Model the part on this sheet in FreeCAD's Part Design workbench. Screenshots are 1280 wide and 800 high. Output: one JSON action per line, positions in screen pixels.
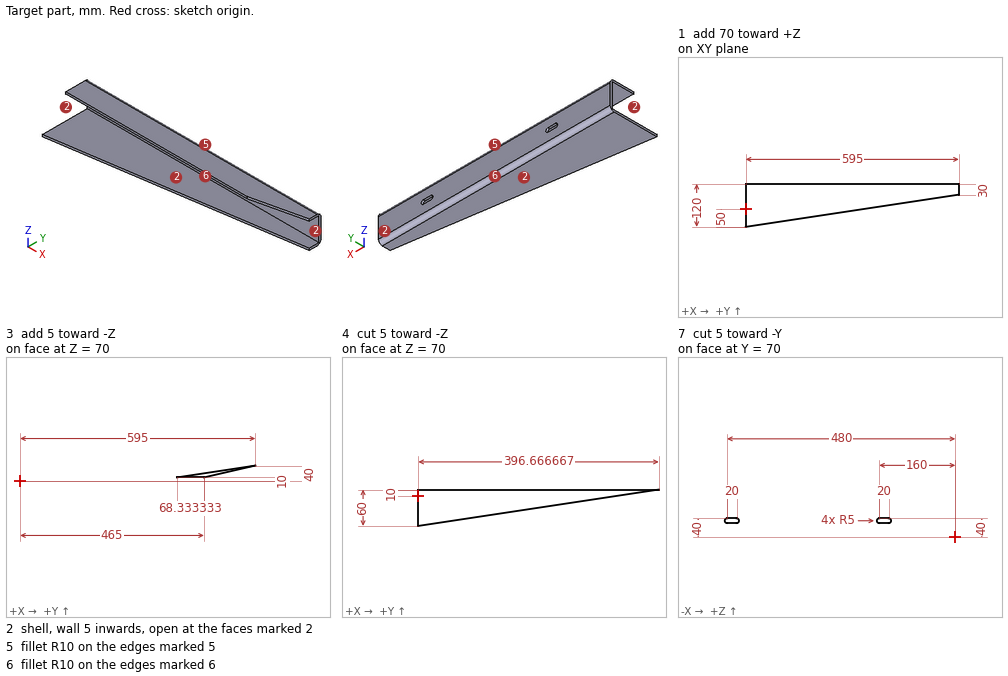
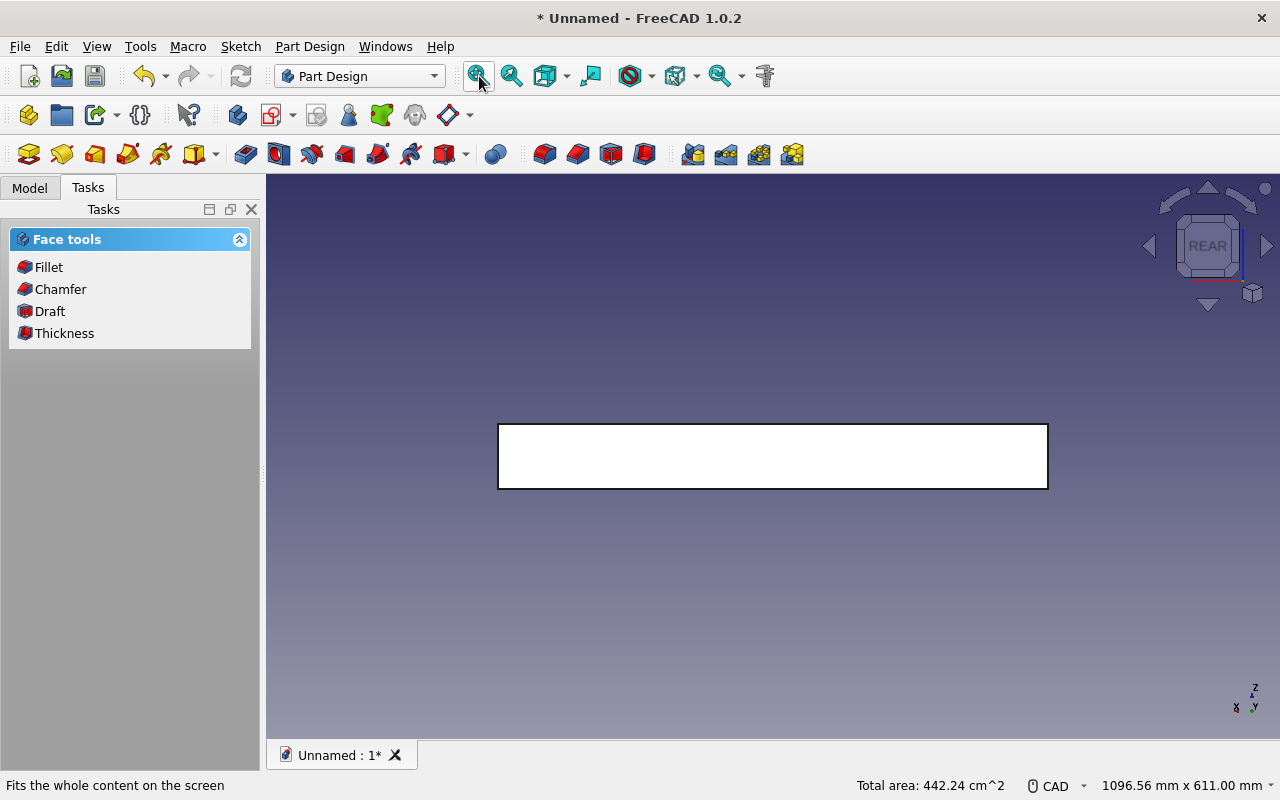
{"action": "key", "text": "6"}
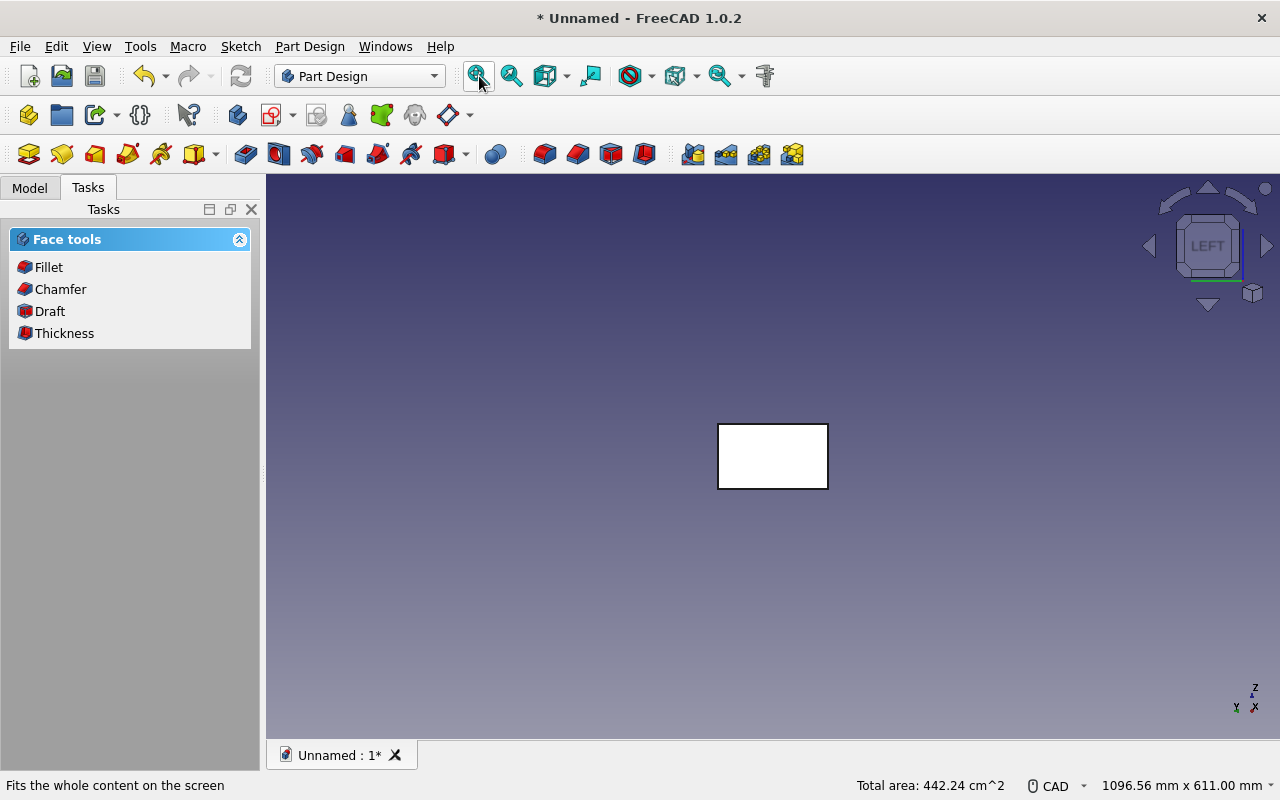
{"action": "key", "text": "v f"}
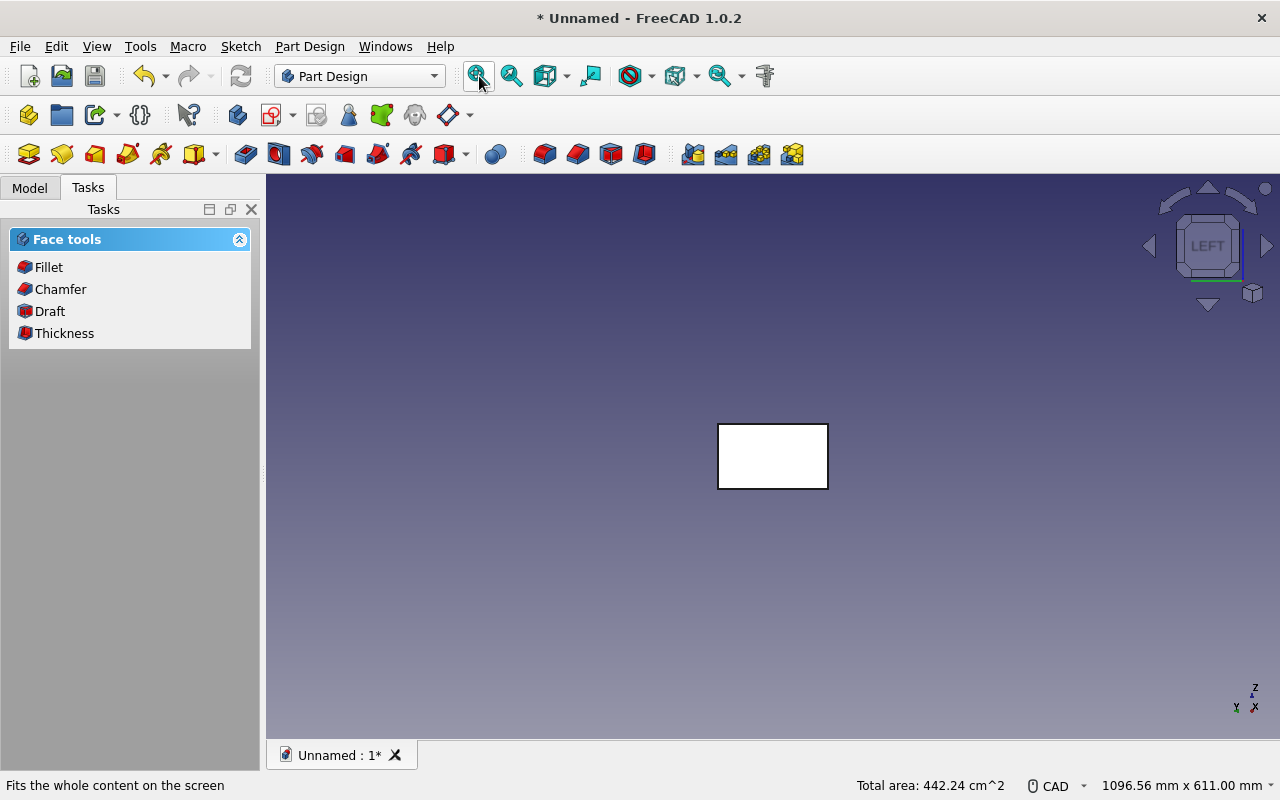
{"action": "left_click", "coordinate": [757, 455], "text": "ctrl"}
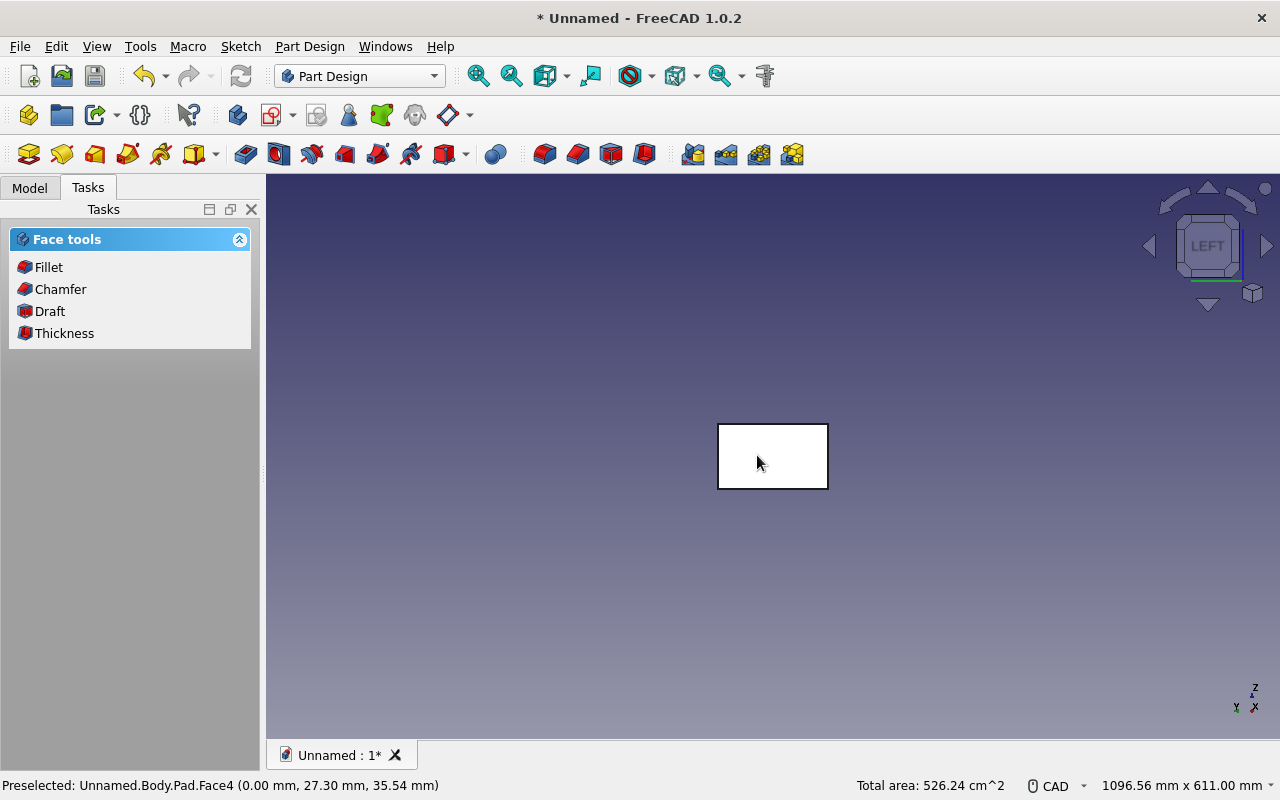
{"action": "left_click", "coordinate": [644, 154]}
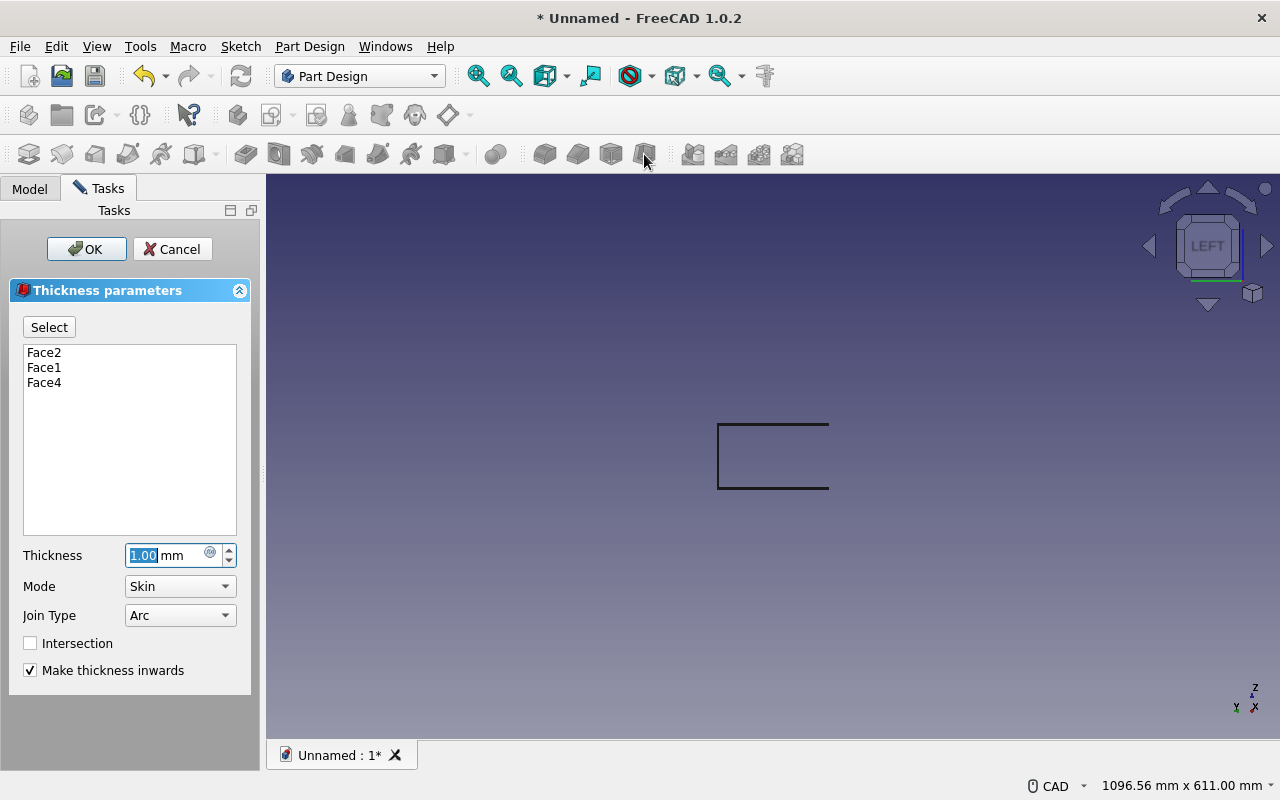
{"action": "type", "text": "5"}
{"action": "key", "text": "Tab"}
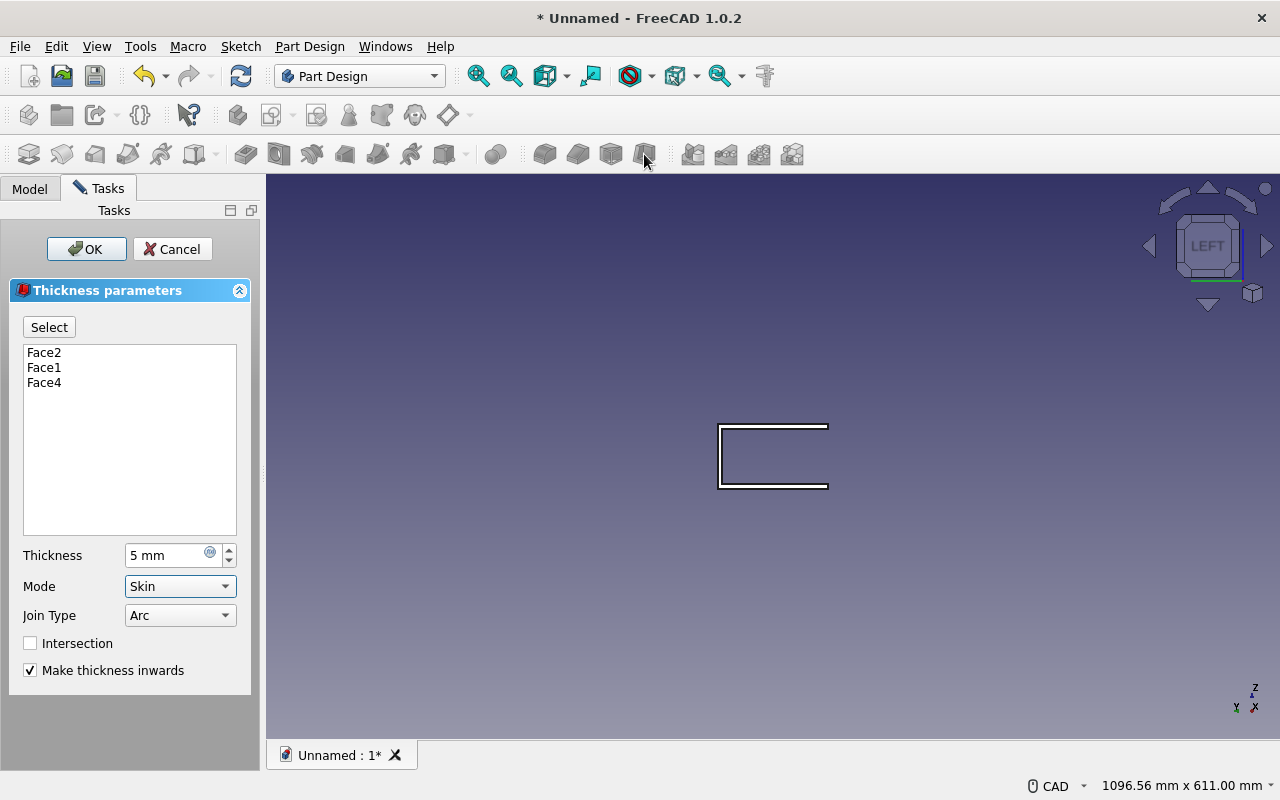
{"action": "left_click", "coordinate": [181, 616]}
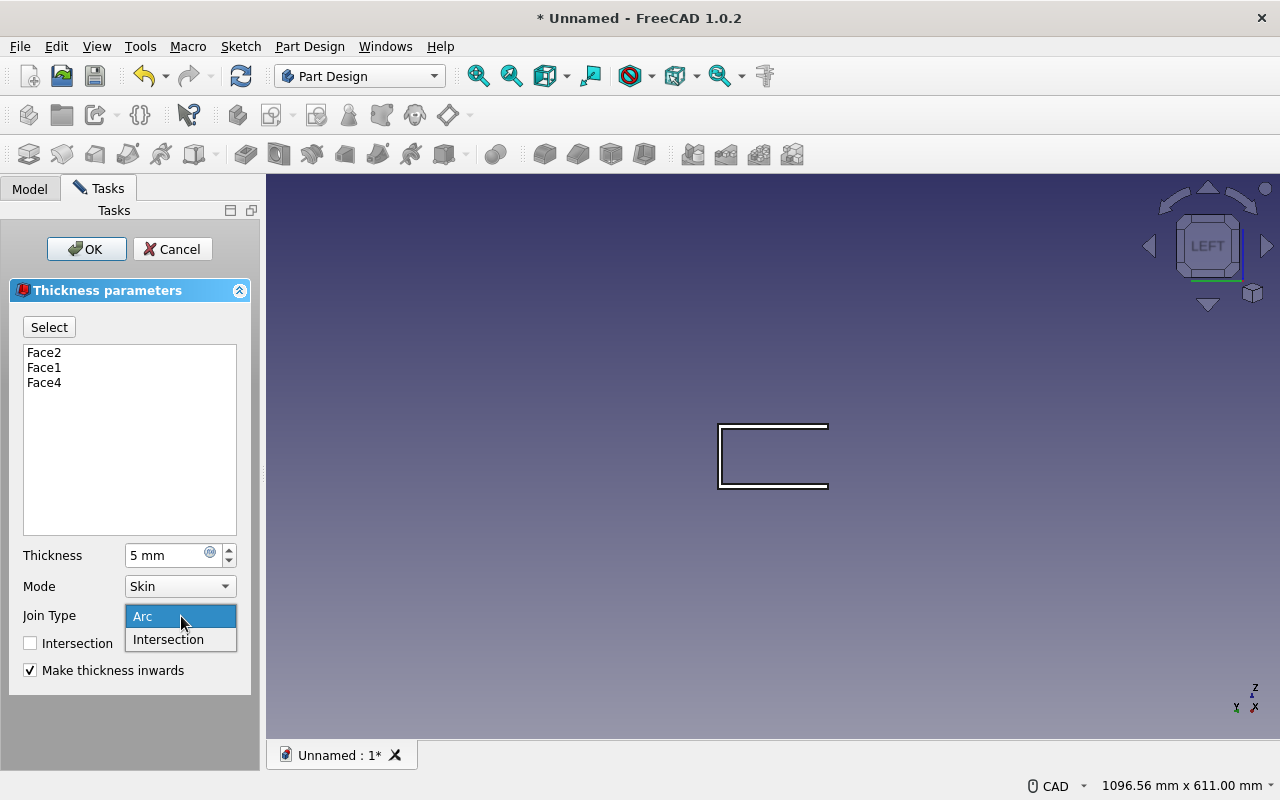
{"action": "left_click", "coordinate": [179, 640]}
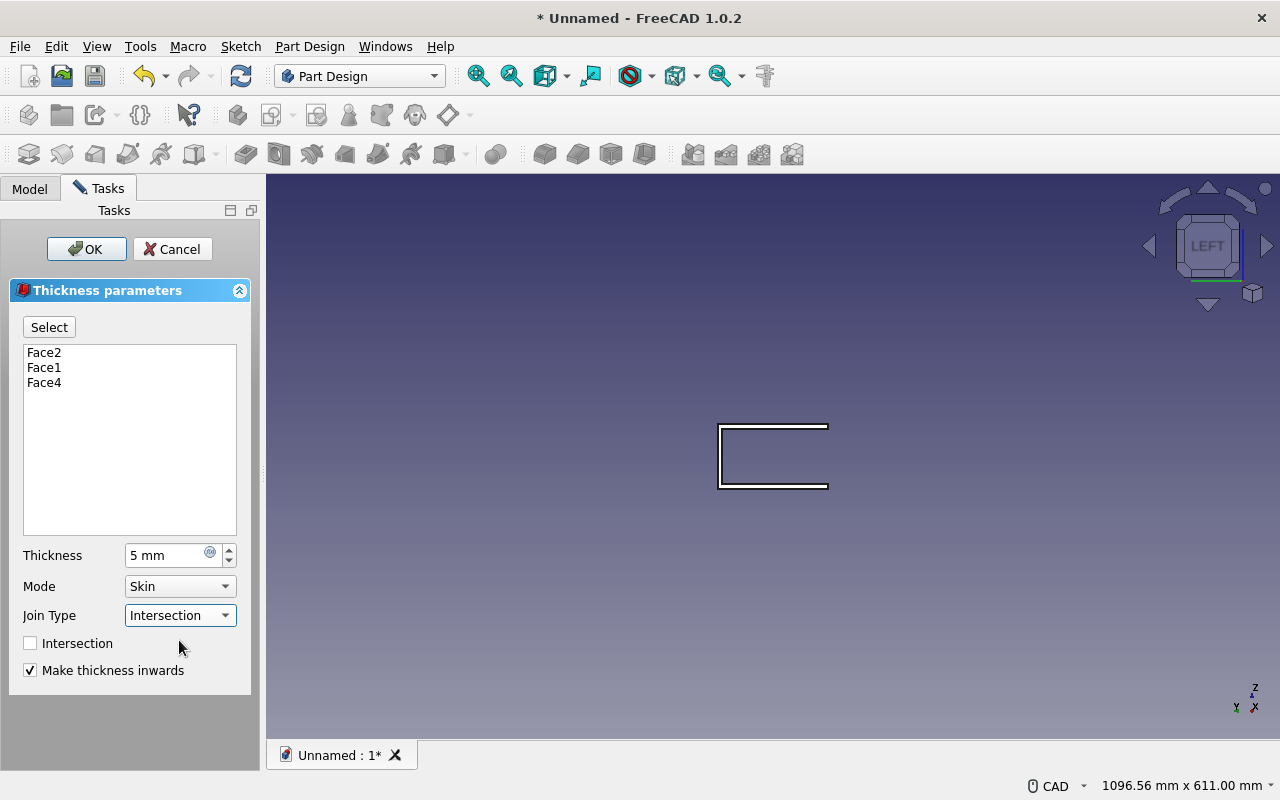
{"action": "left_click", "coordinate": [87, 249]}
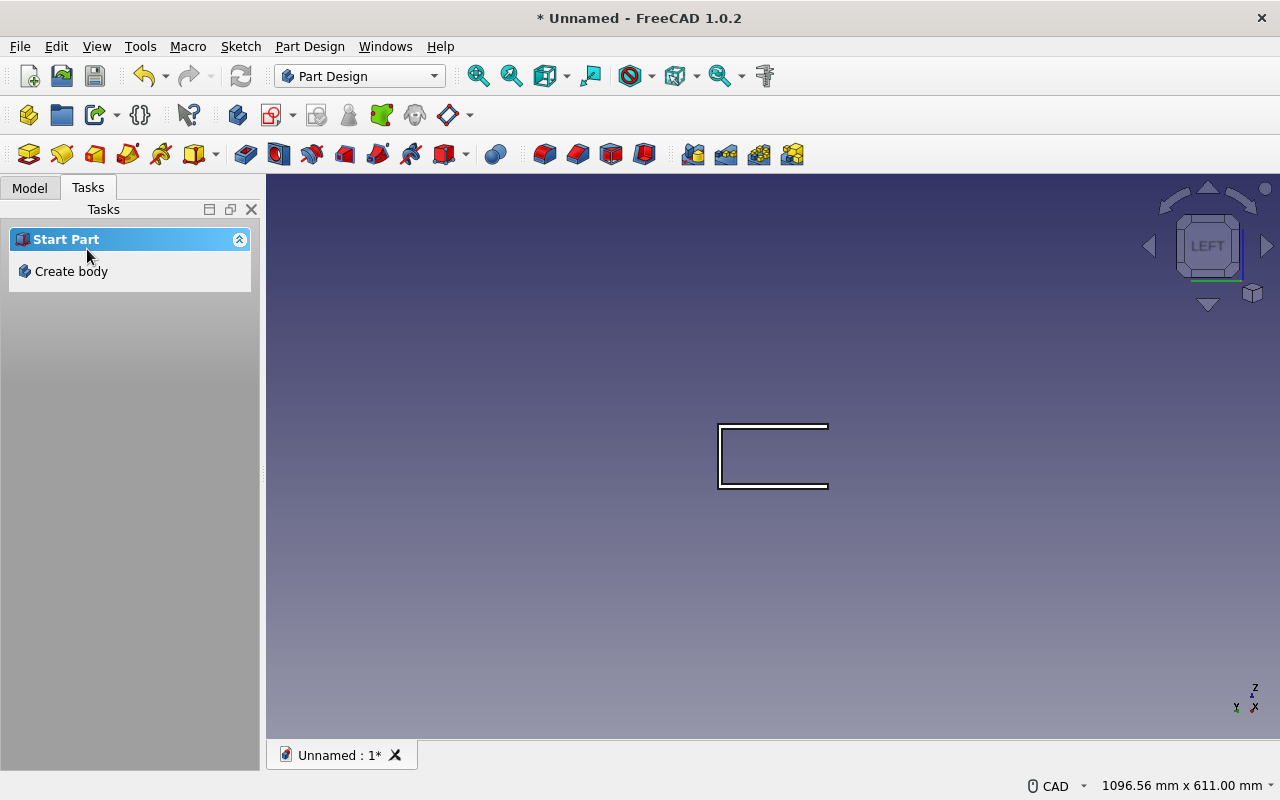
{"action": "left_click", "coordinate": [479, 76]}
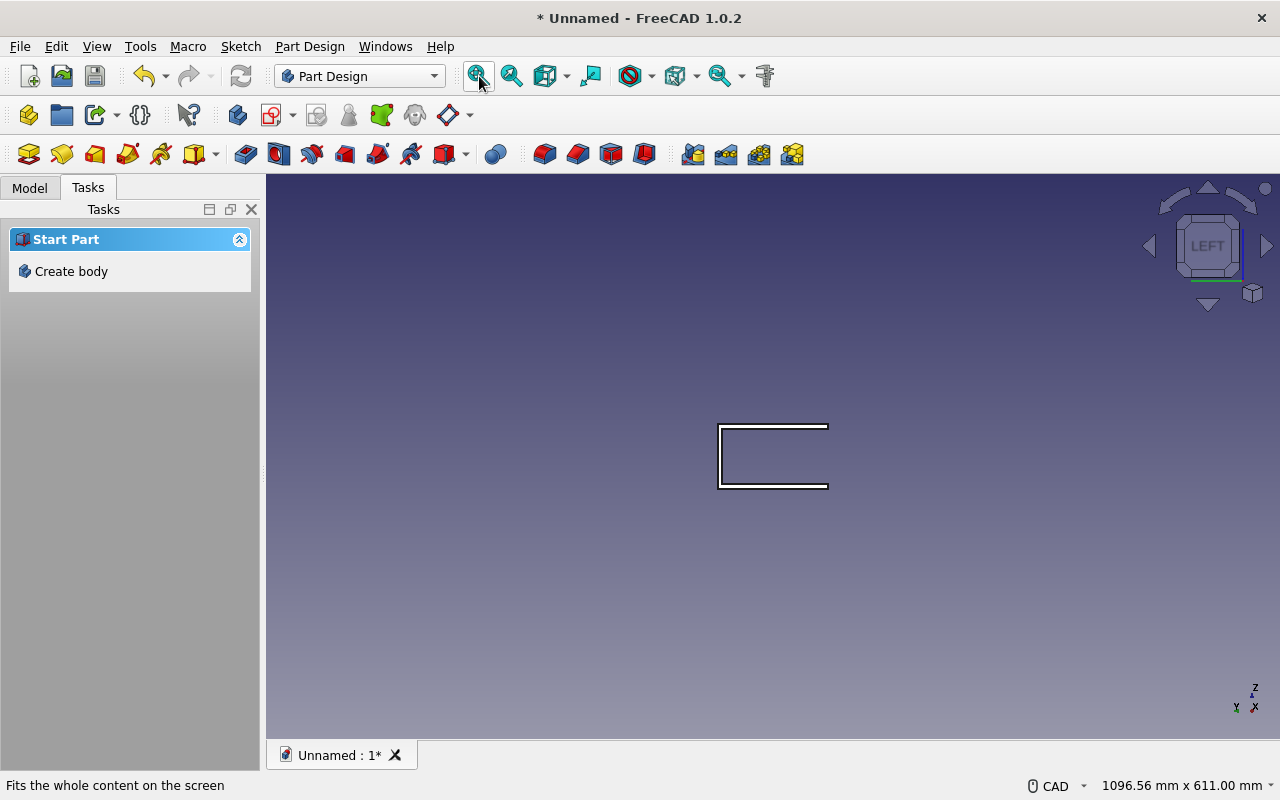
{"action": "key", "text": "0"}